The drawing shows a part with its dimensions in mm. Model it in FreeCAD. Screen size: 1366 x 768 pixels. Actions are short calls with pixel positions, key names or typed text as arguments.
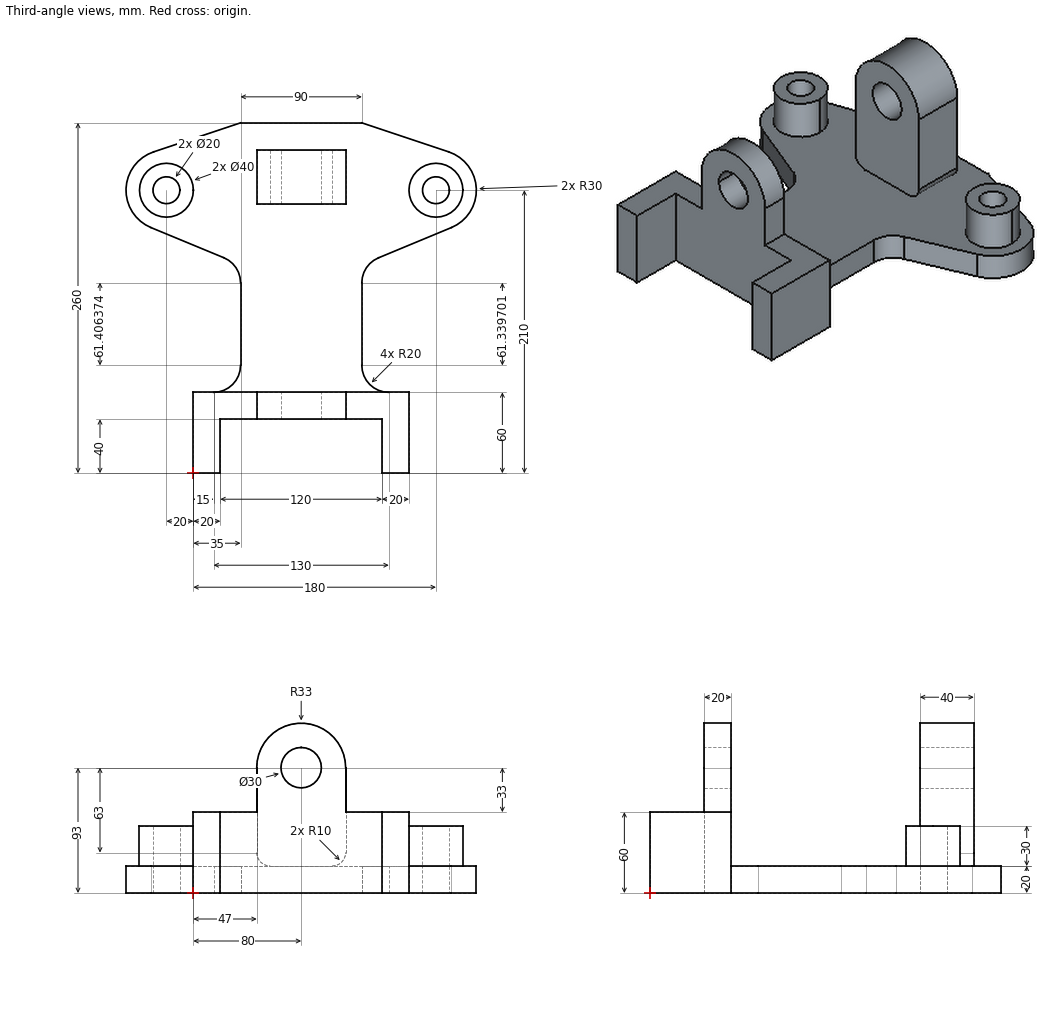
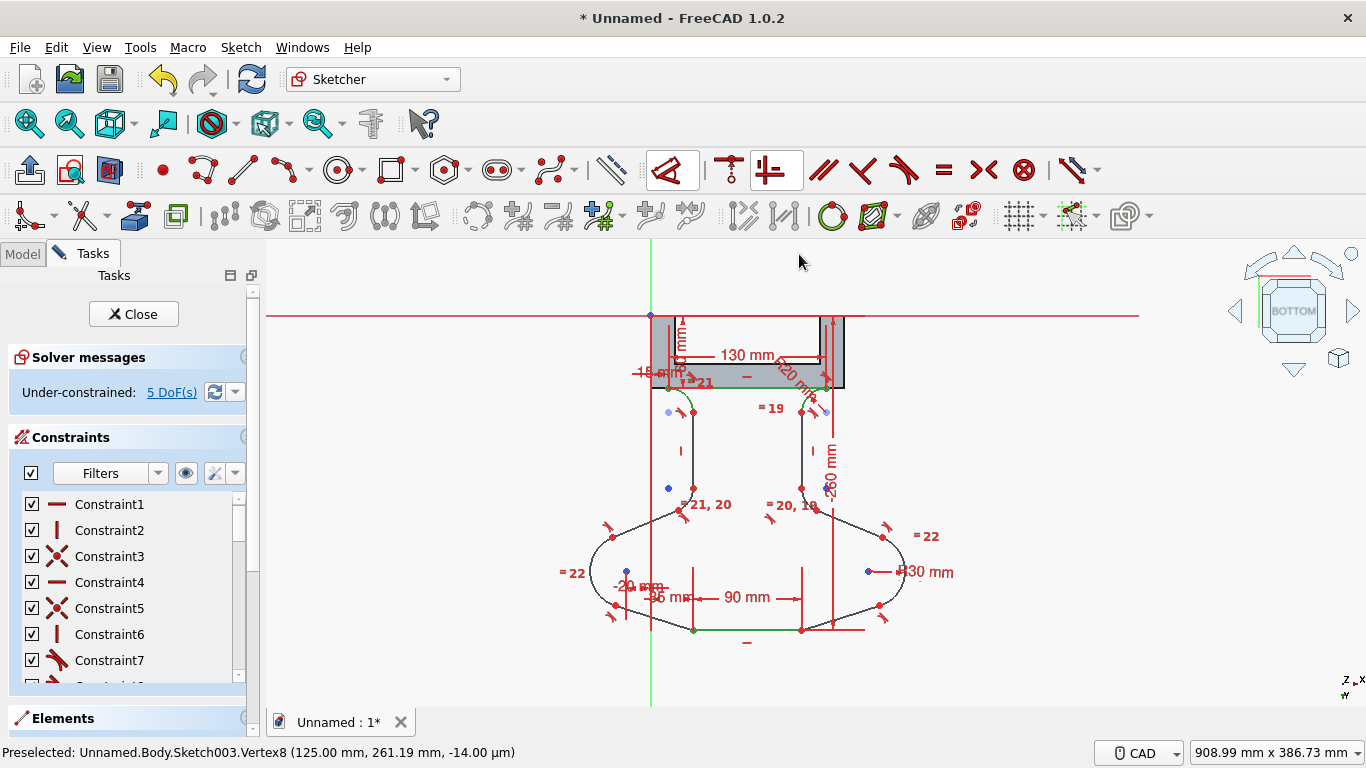
click(869, 571)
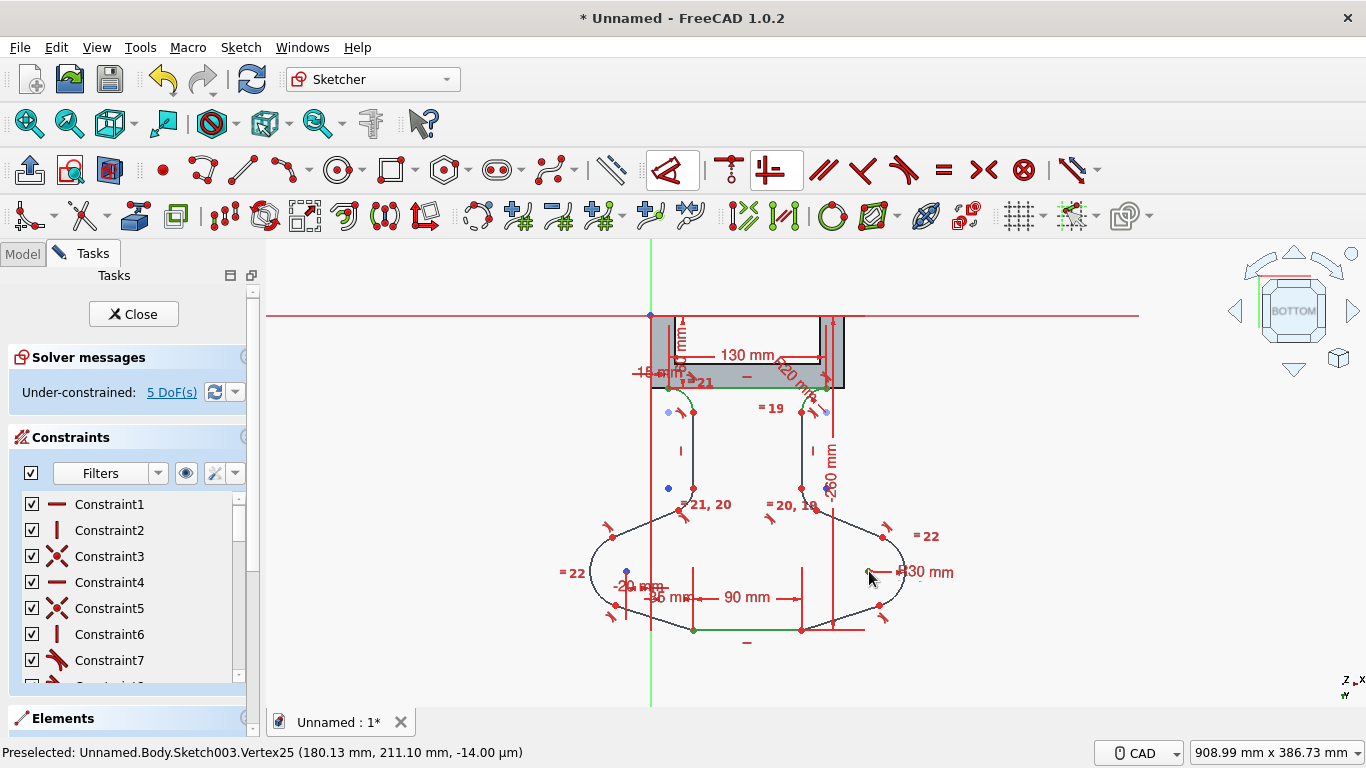
click(694, 170)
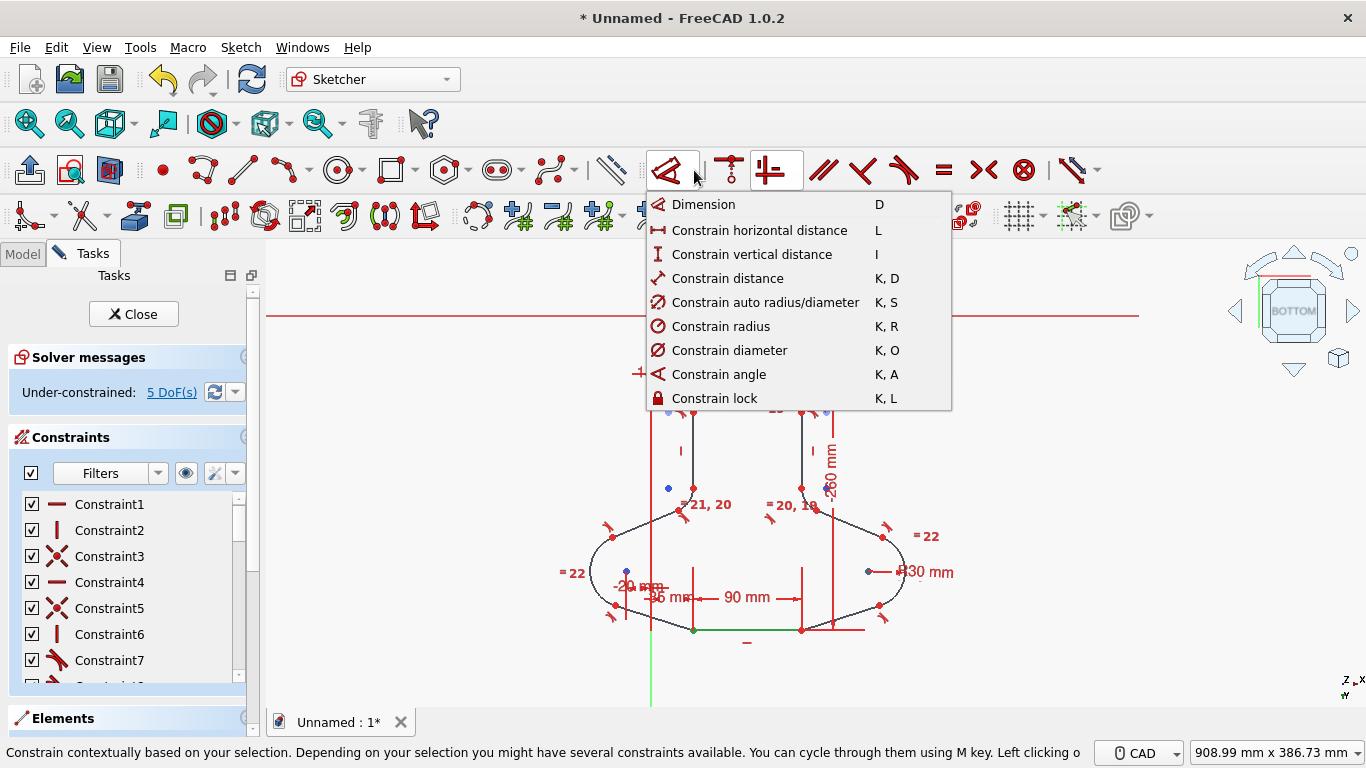
click(799, 230)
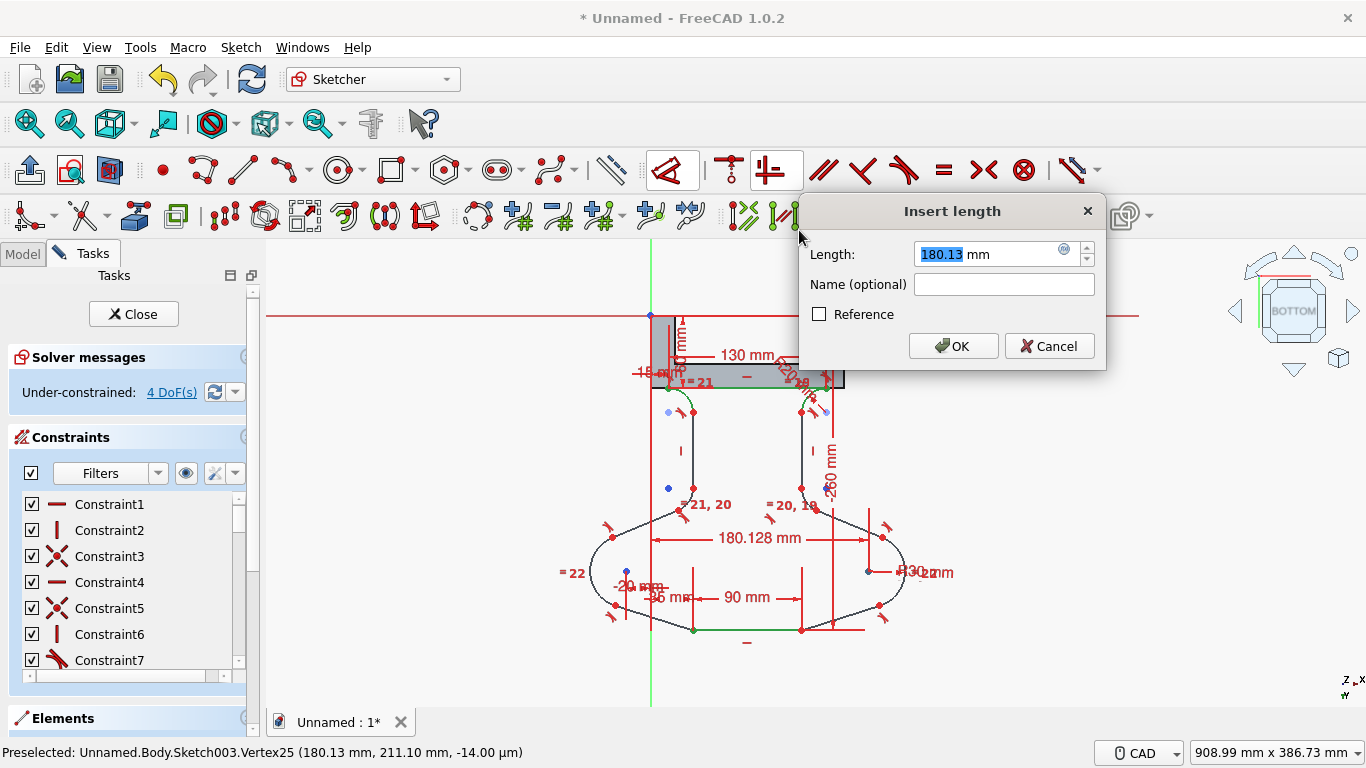
text(180)
key(Return)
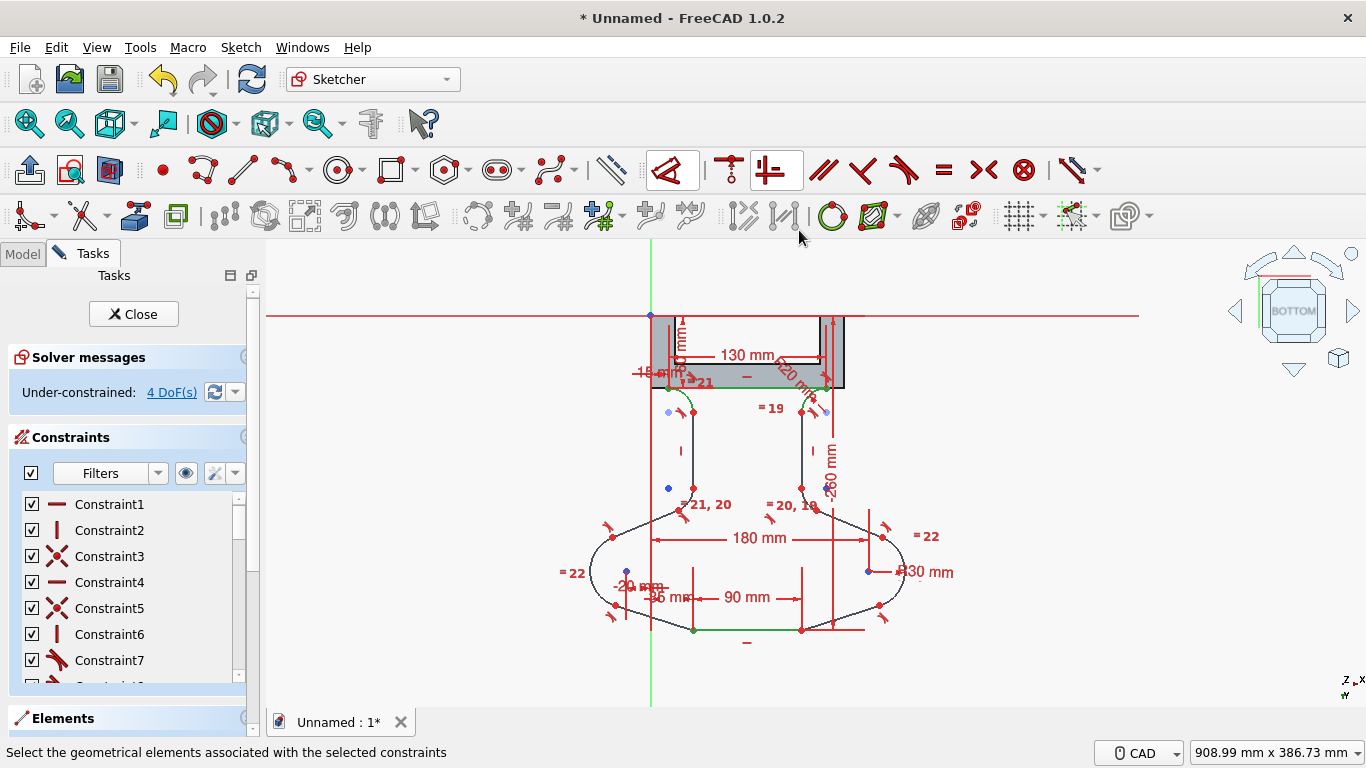
click(869, 571)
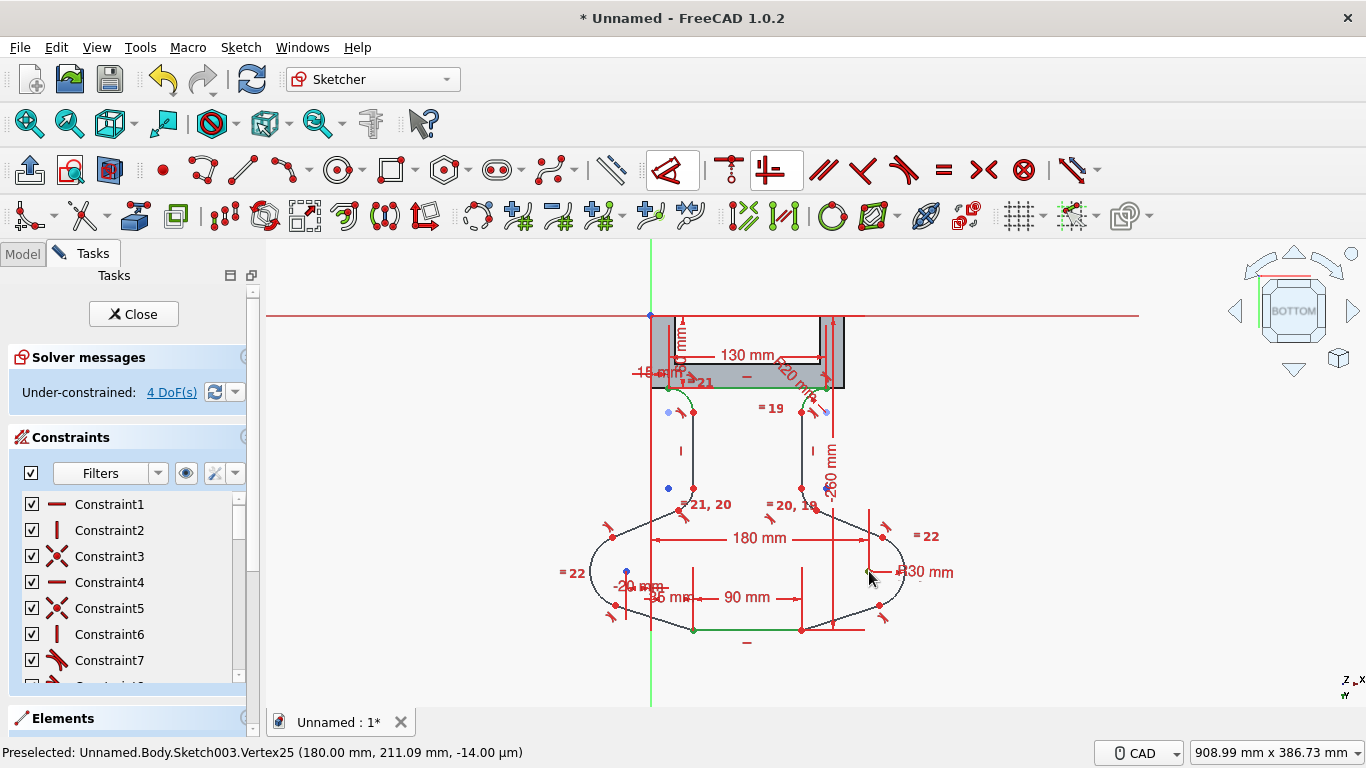
key(i)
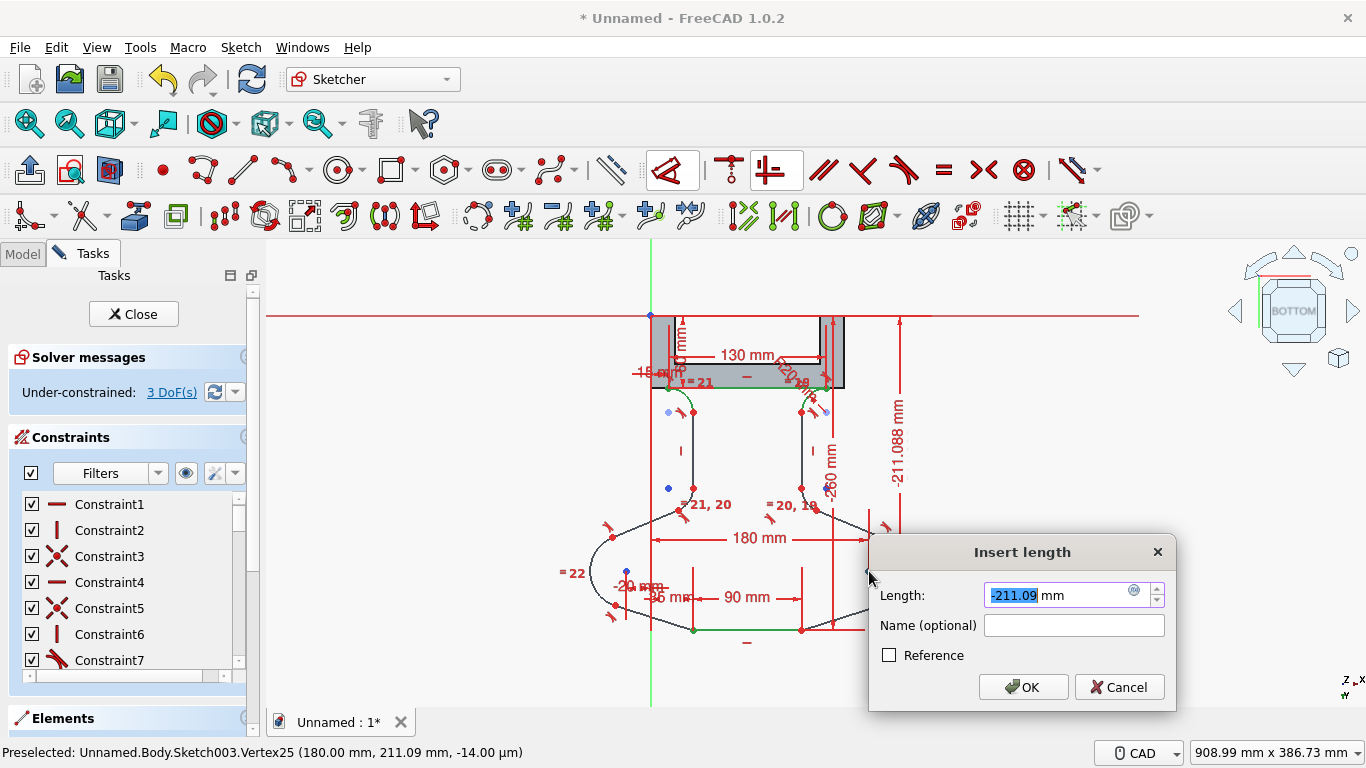
text(-210)
key(Return)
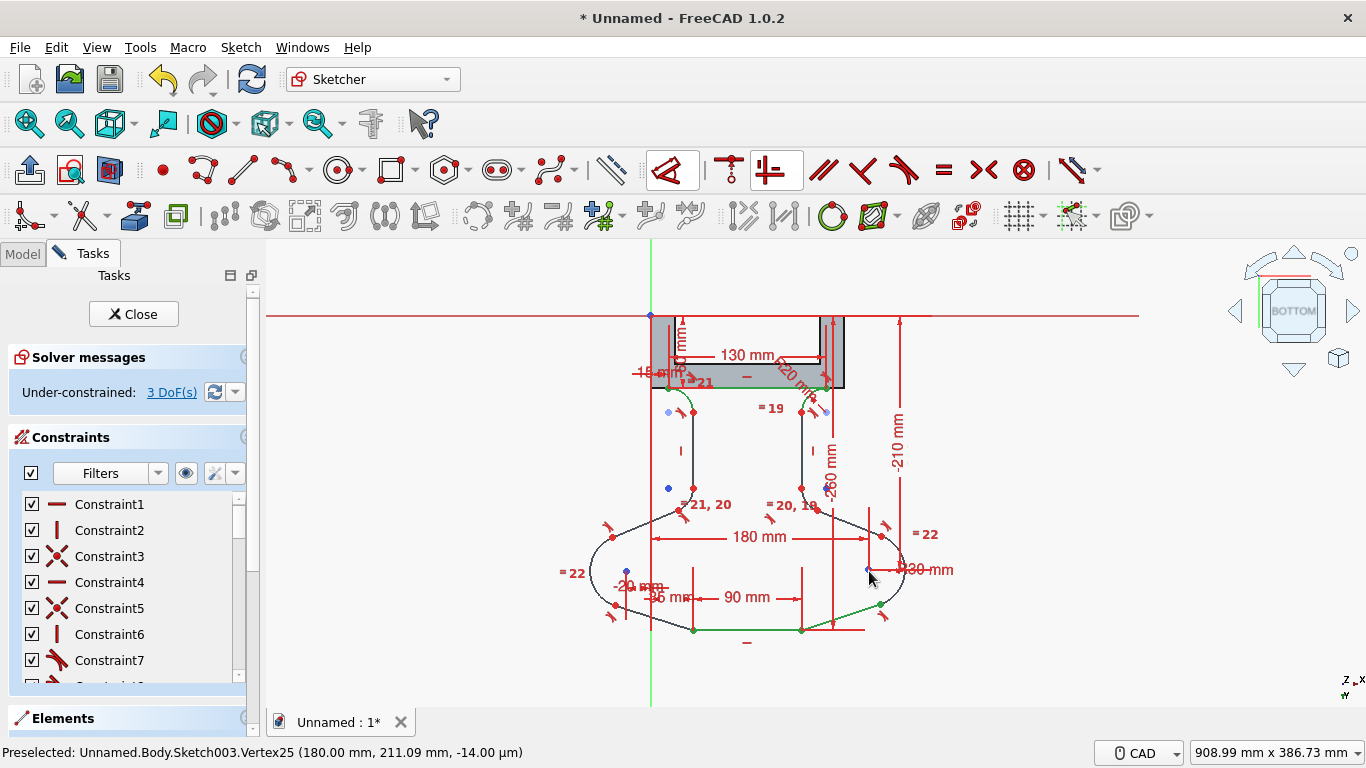
click(626, 571)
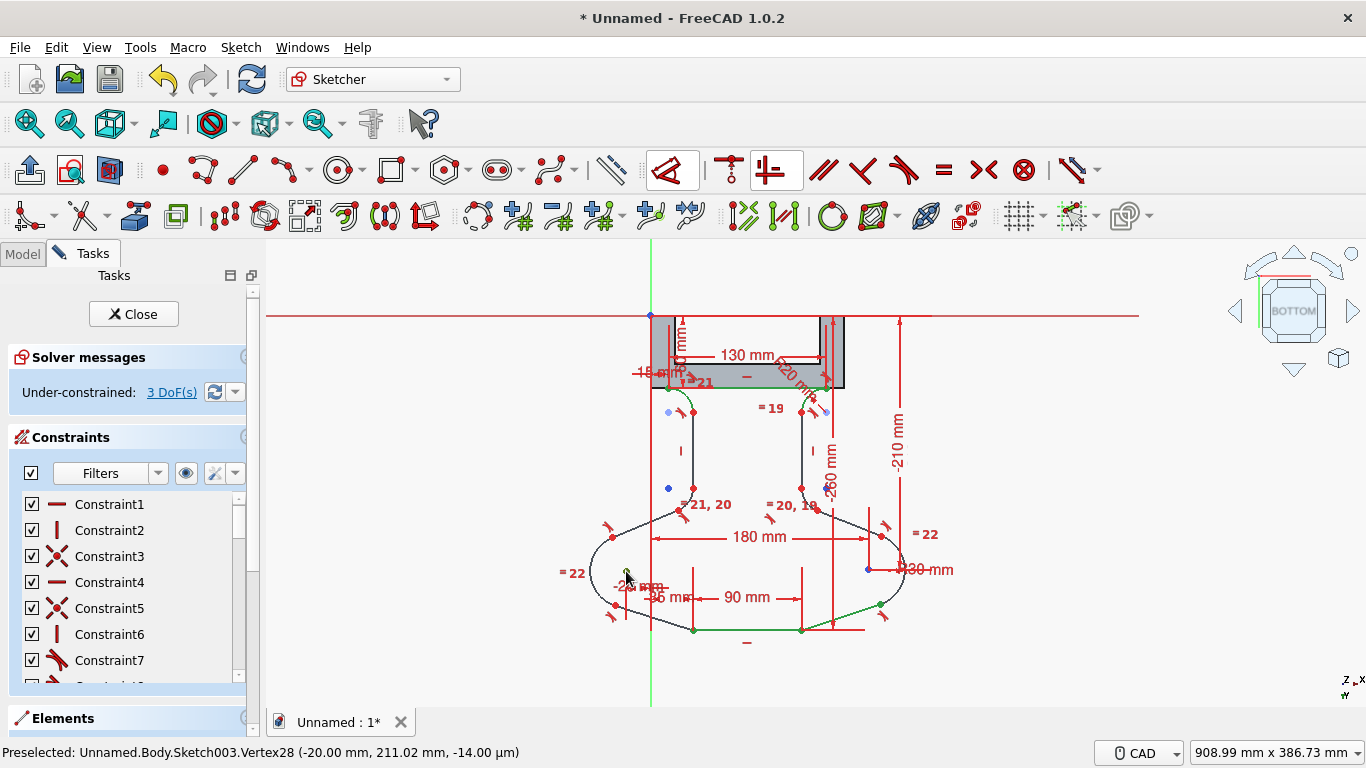
key(i)